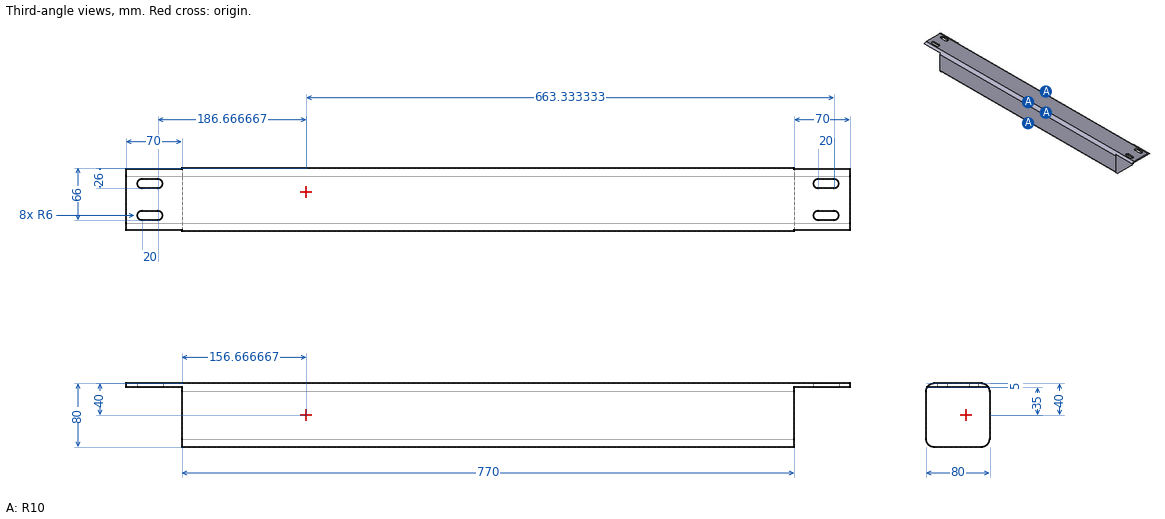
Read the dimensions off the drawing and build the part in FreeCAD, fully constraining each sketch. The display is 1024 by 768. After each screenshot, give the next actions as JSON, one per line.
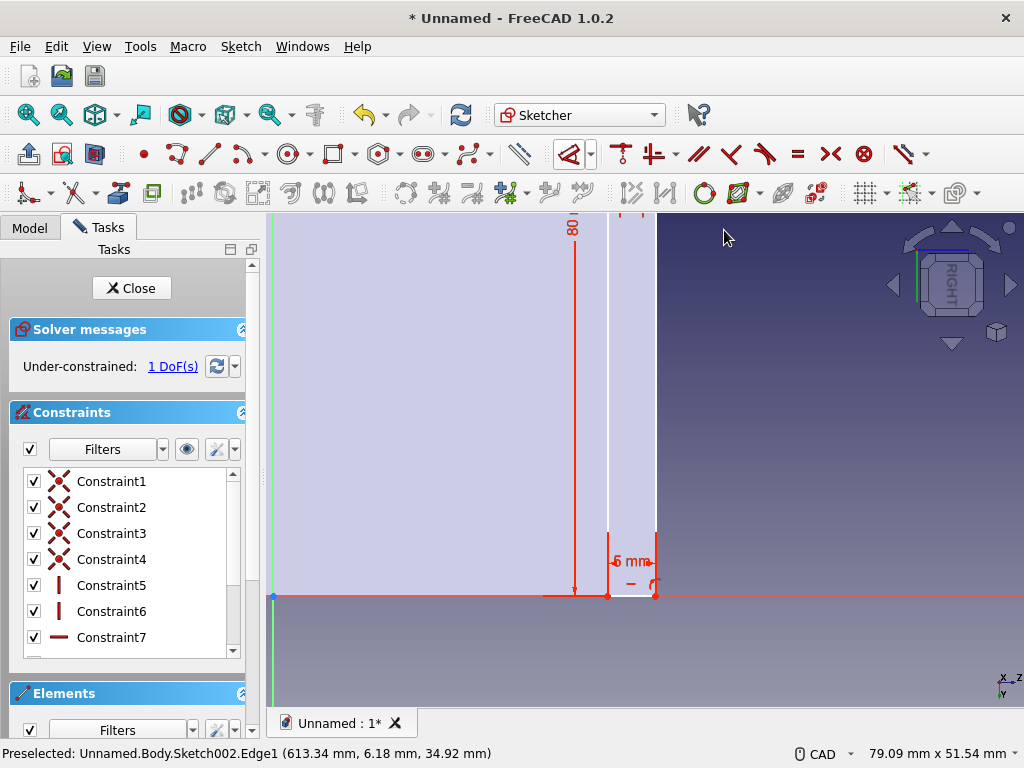
{"action": "scroll", "coordinate": [642, 604], "scroll_direction": "down", "scroll_amount": 5}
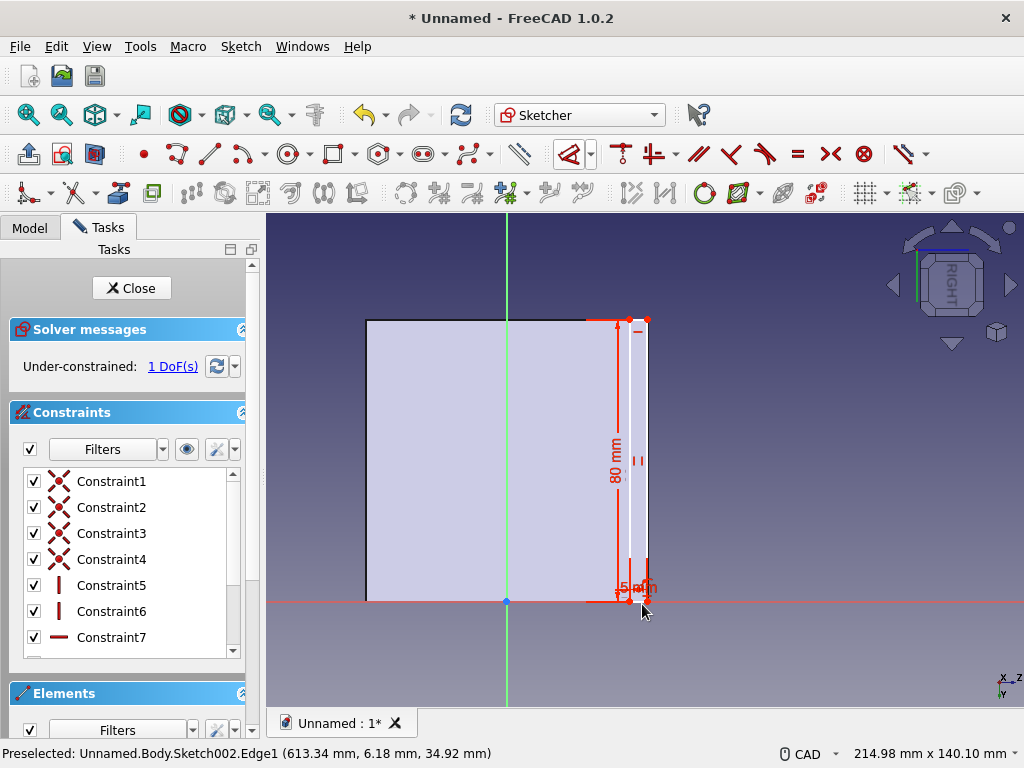
{"action": "left_click", "coordinate": [630, 320]}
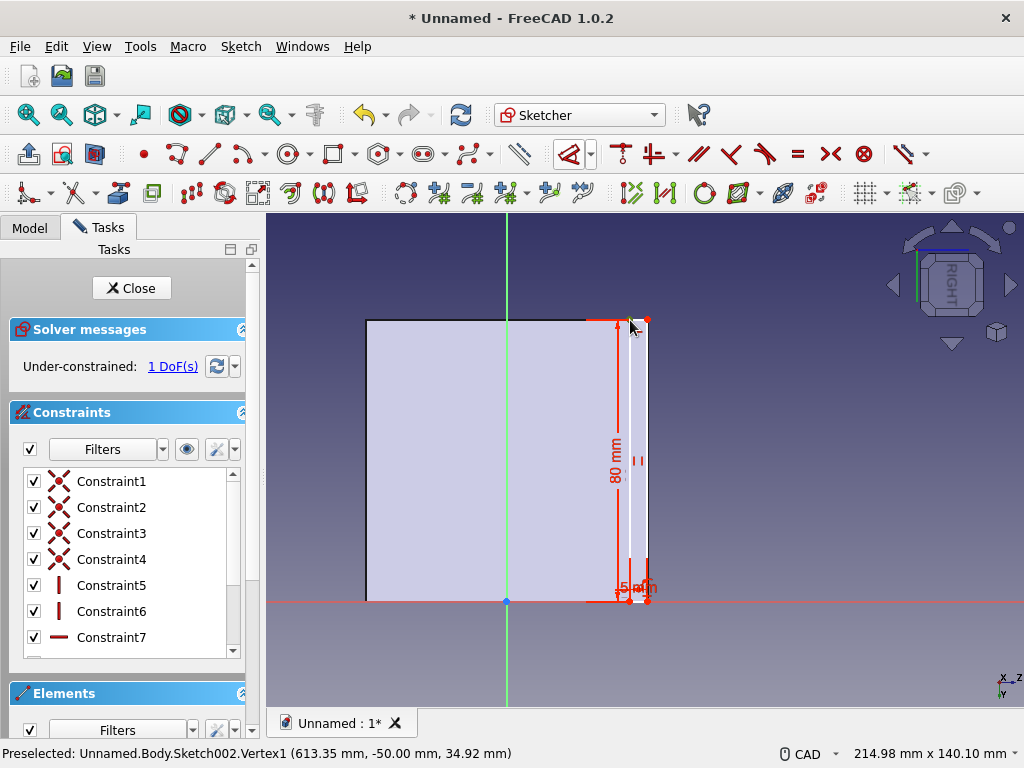
{"action": "left_click", "coordinate": [590, 154]}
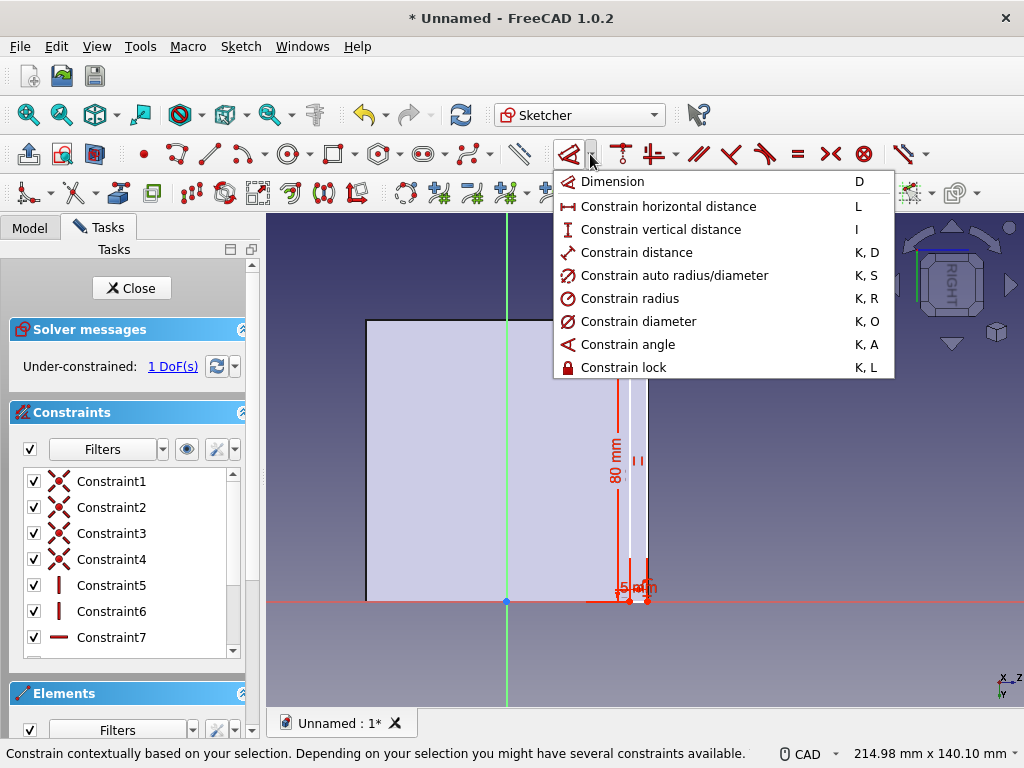
{"action": "left_click", "coordinate": [724, 206]}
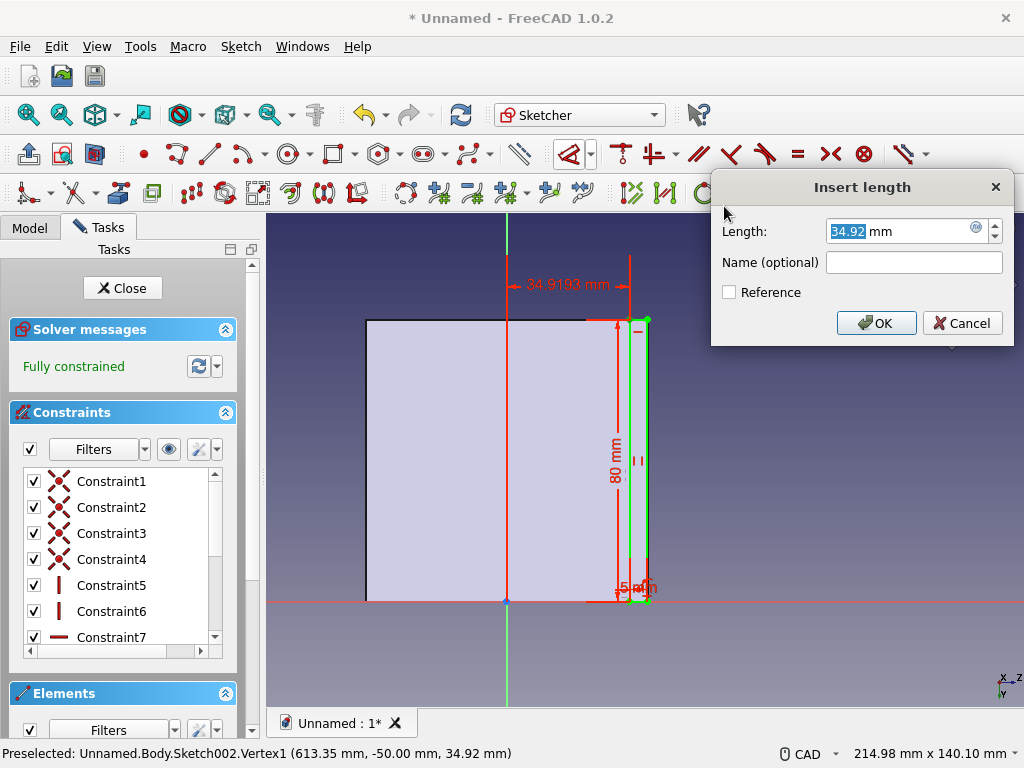
{"action": "type", "text": "35"}
{"action": "key", "text": "Return"}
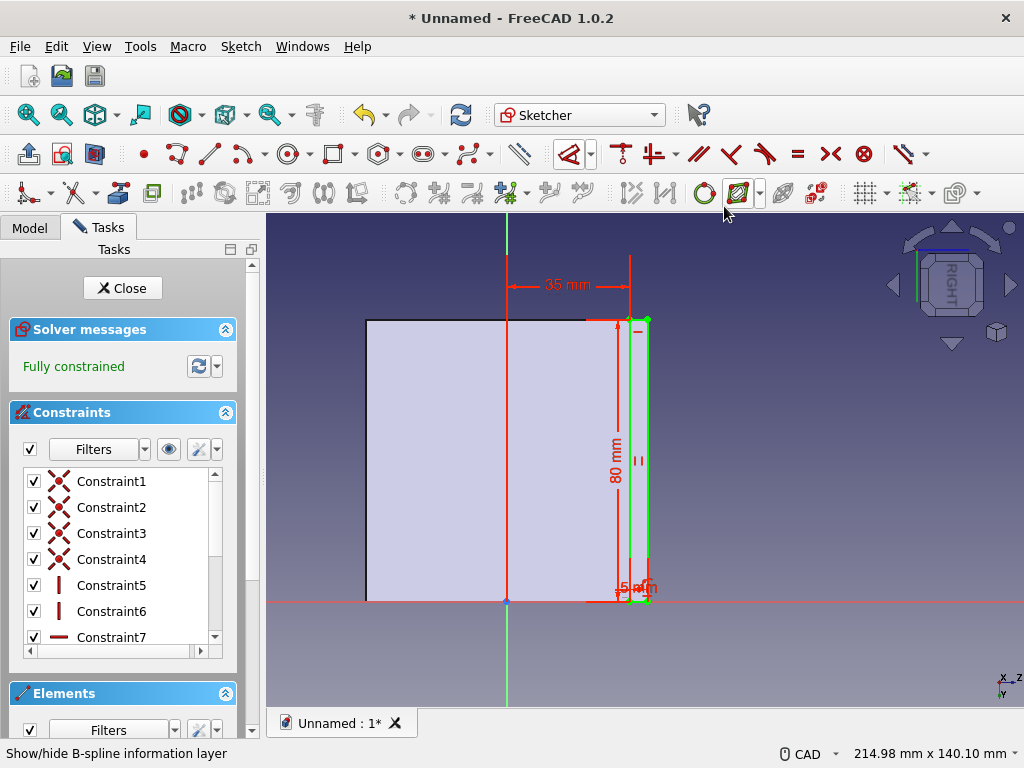
{"action": "left_click", "coordinate": [123, 288]}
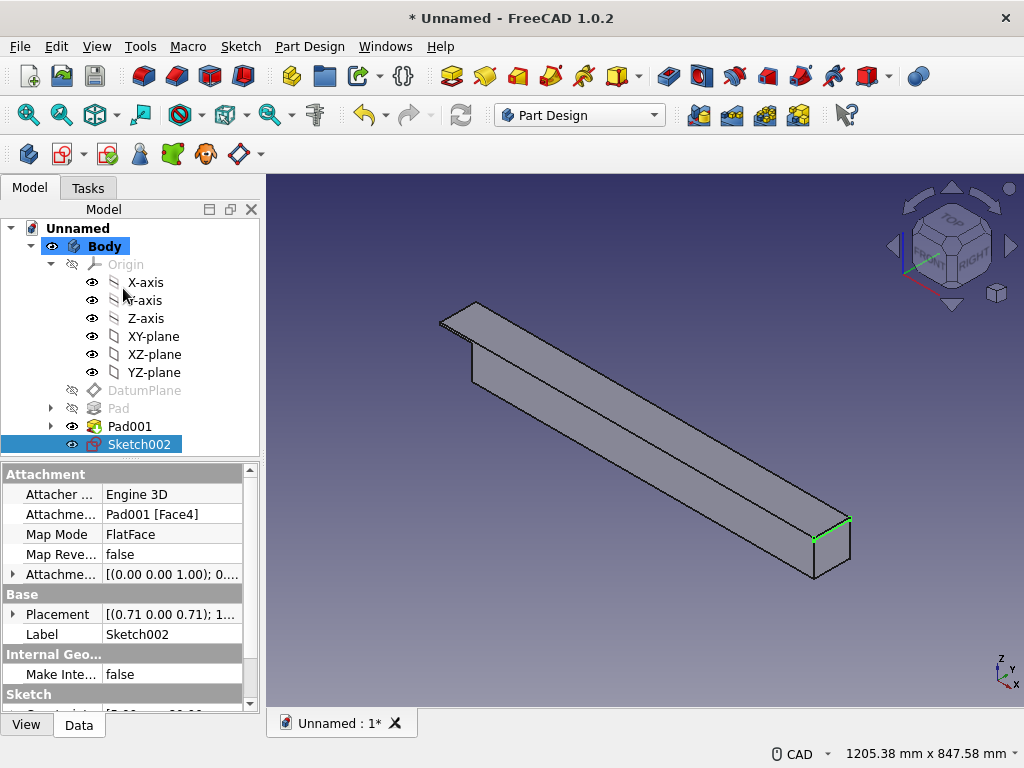
{"action": "left_click", "coordinate": [452, 76]}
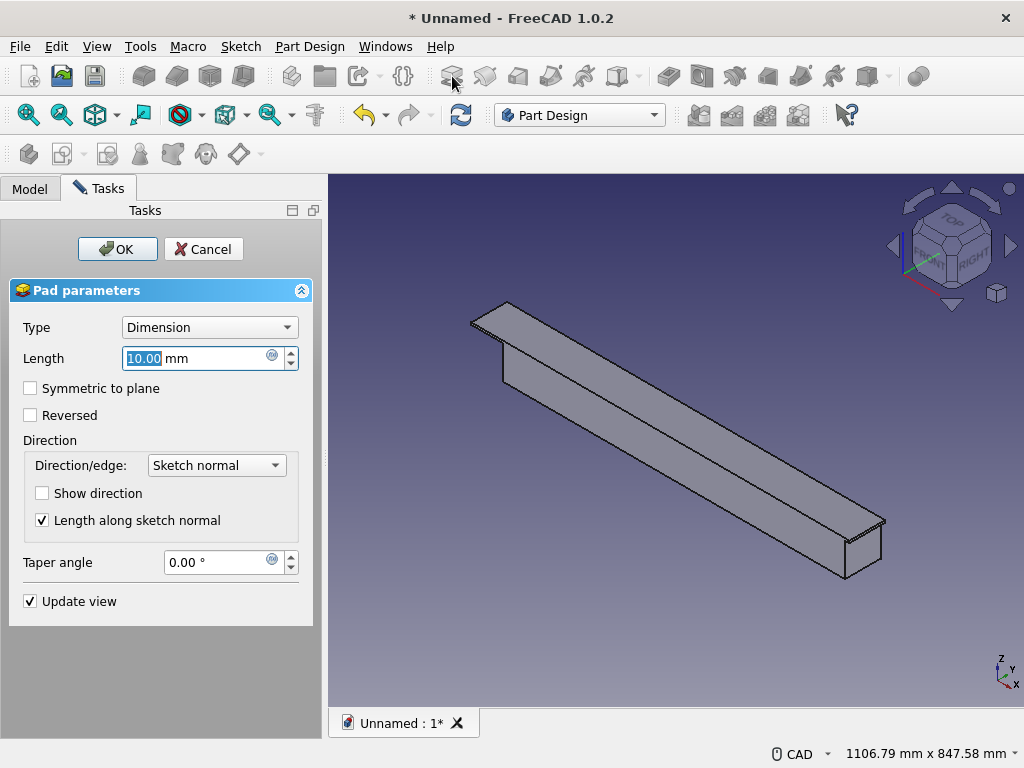
{"action": "type", "text": "70"}
{"action": "key", "text": "Tab"}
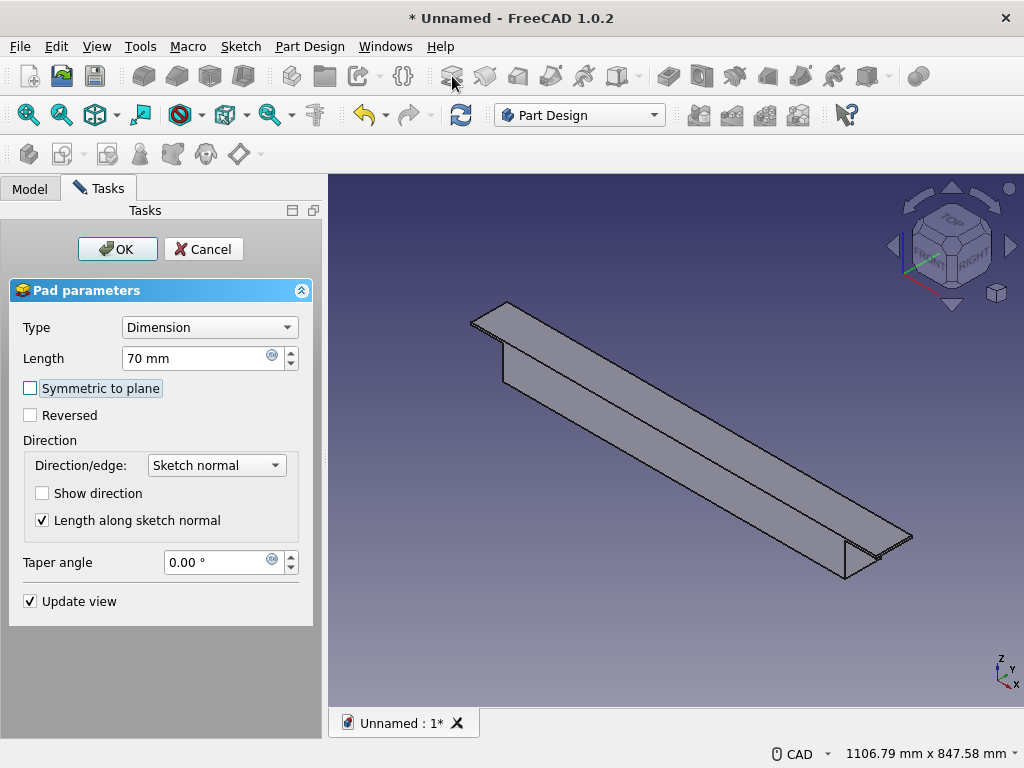
{"action": "left_click", "coordinate": [118, 249]}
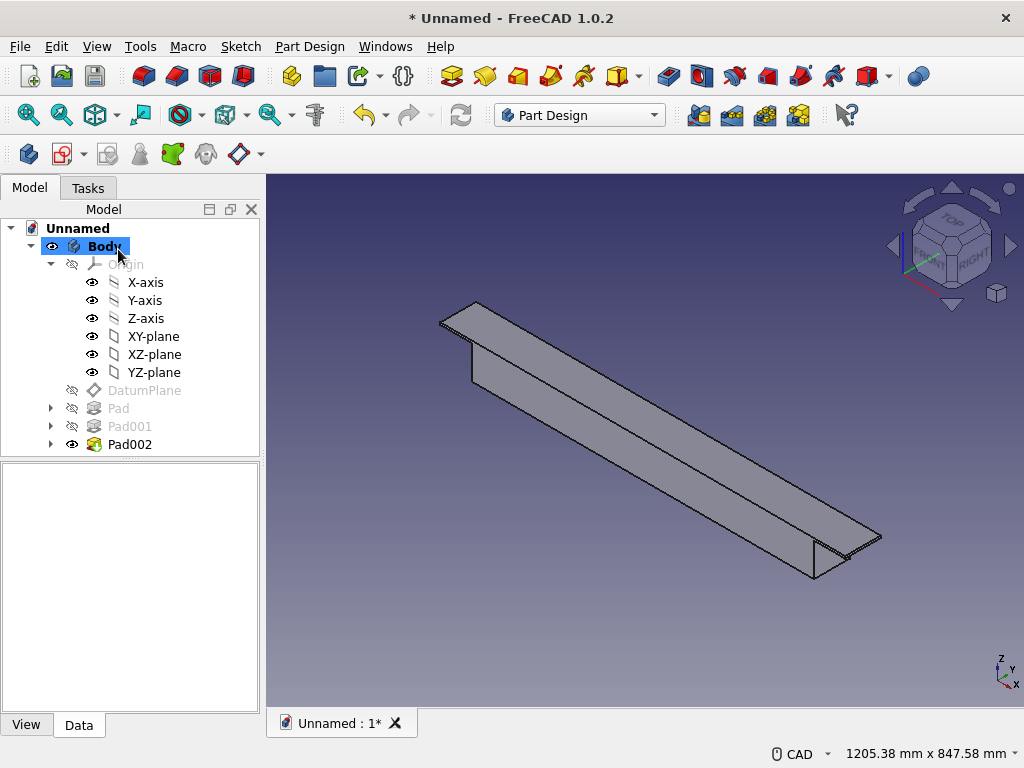
{"action": "left_click", "coordinate": [643, 438]}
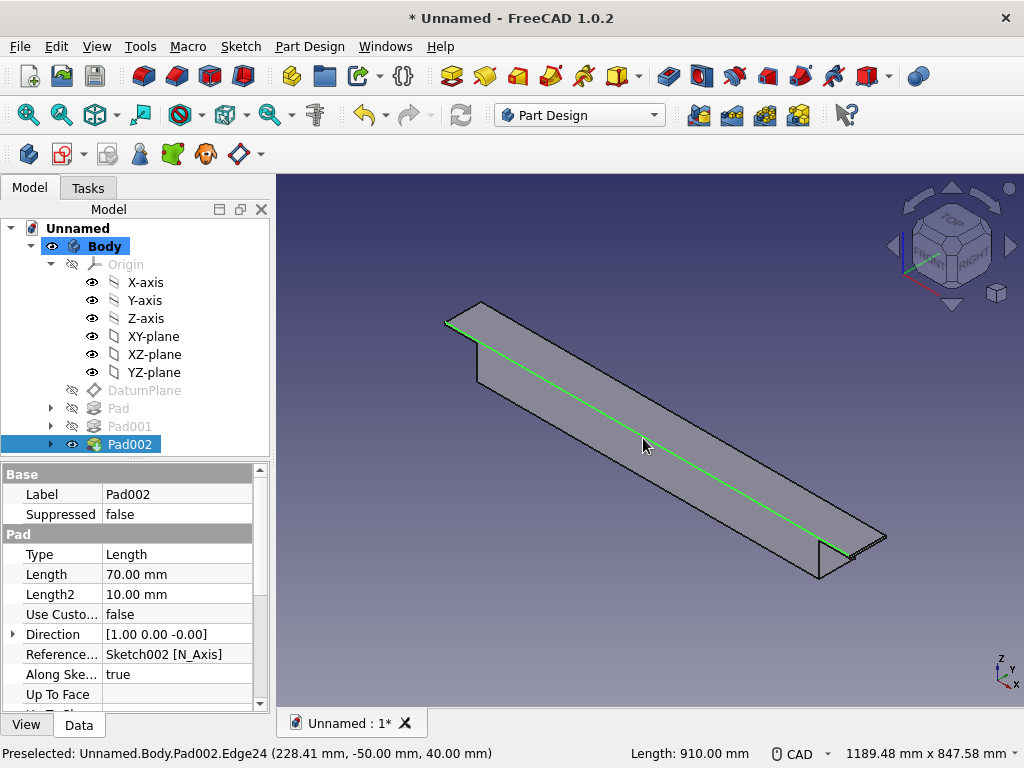
{"action": "key", "text": "2"}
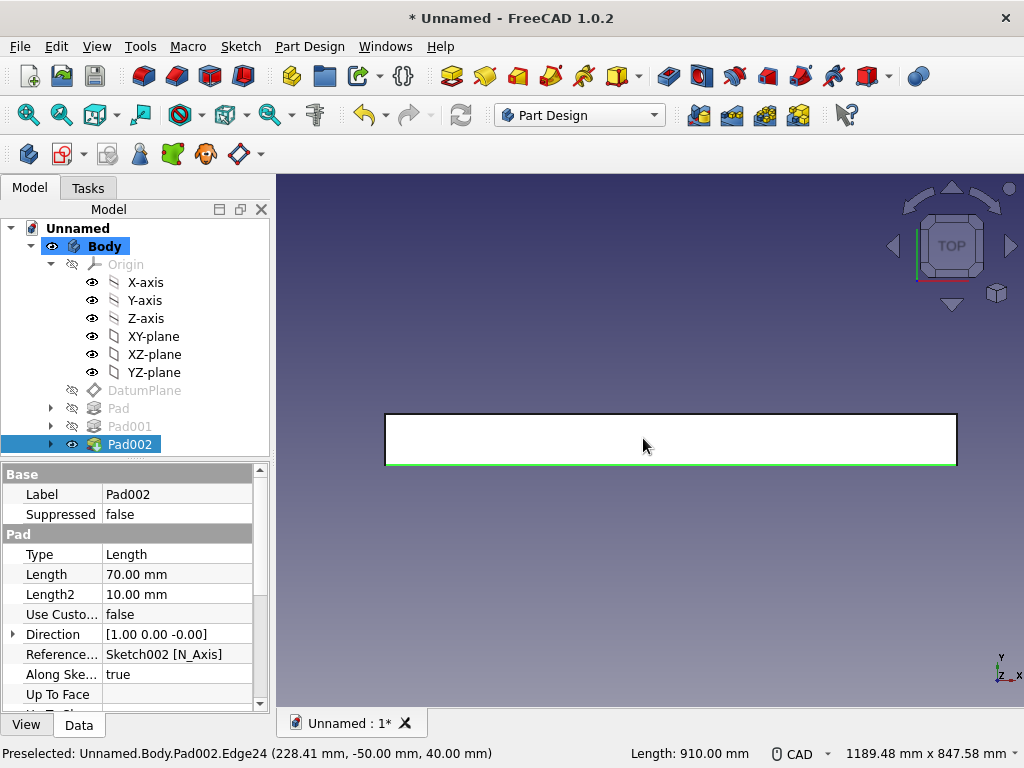
{"action": "left_click", "coordinate": [671, 413], "text": "ctrl"}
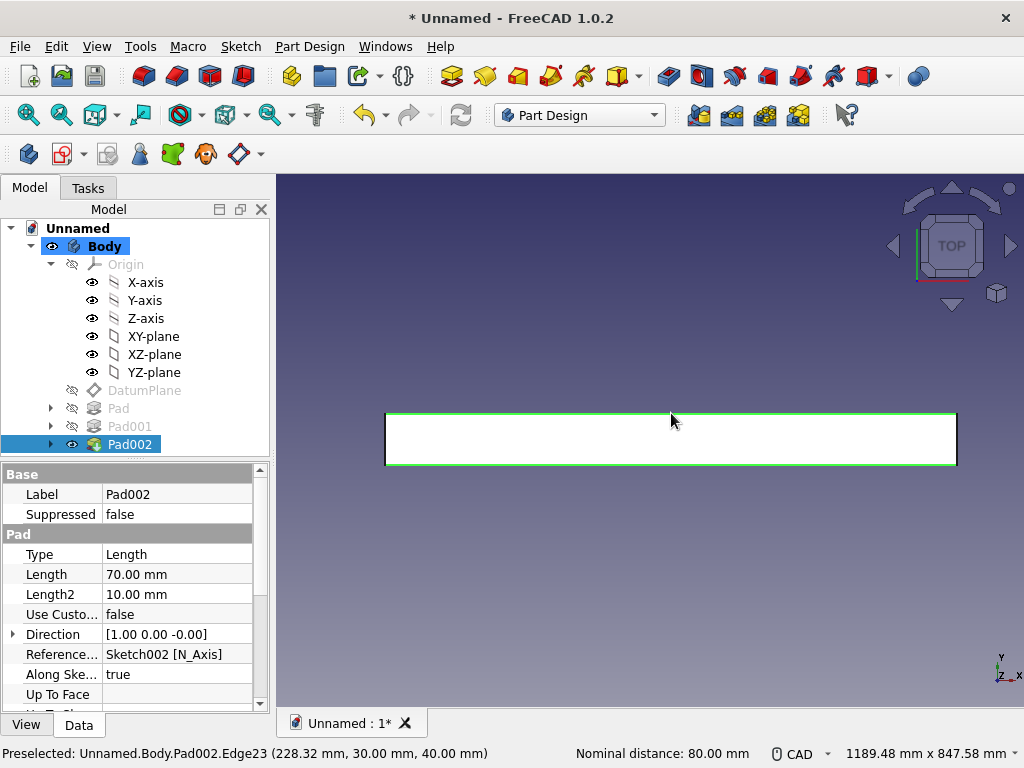
{"action": "key", "text": "0"}